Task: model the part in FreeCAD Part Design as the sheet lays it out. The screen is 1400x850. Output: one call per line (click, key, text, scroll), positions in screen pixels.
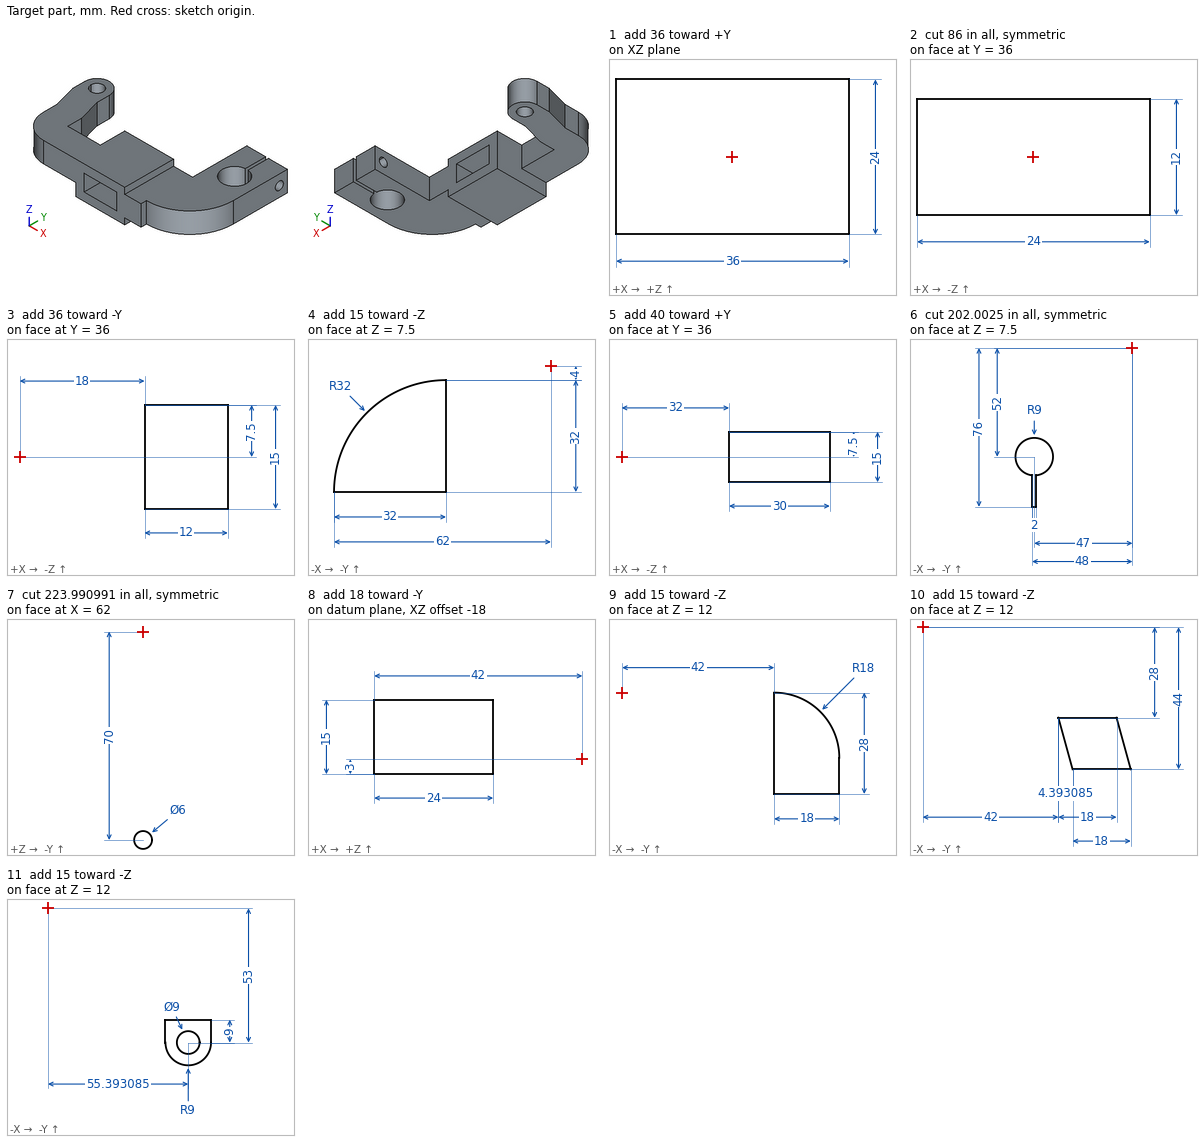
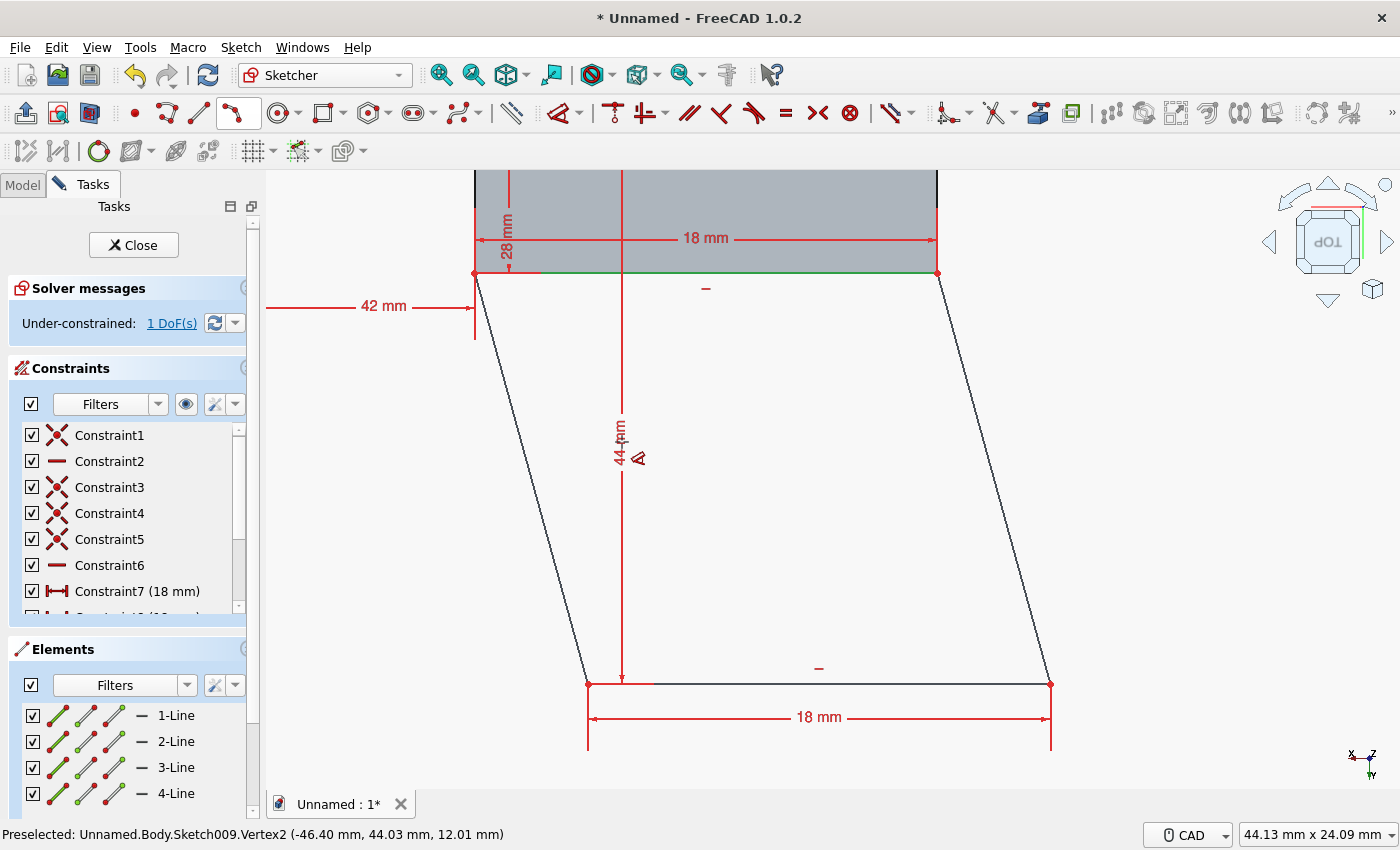
click(509, 396)
click(531, 718)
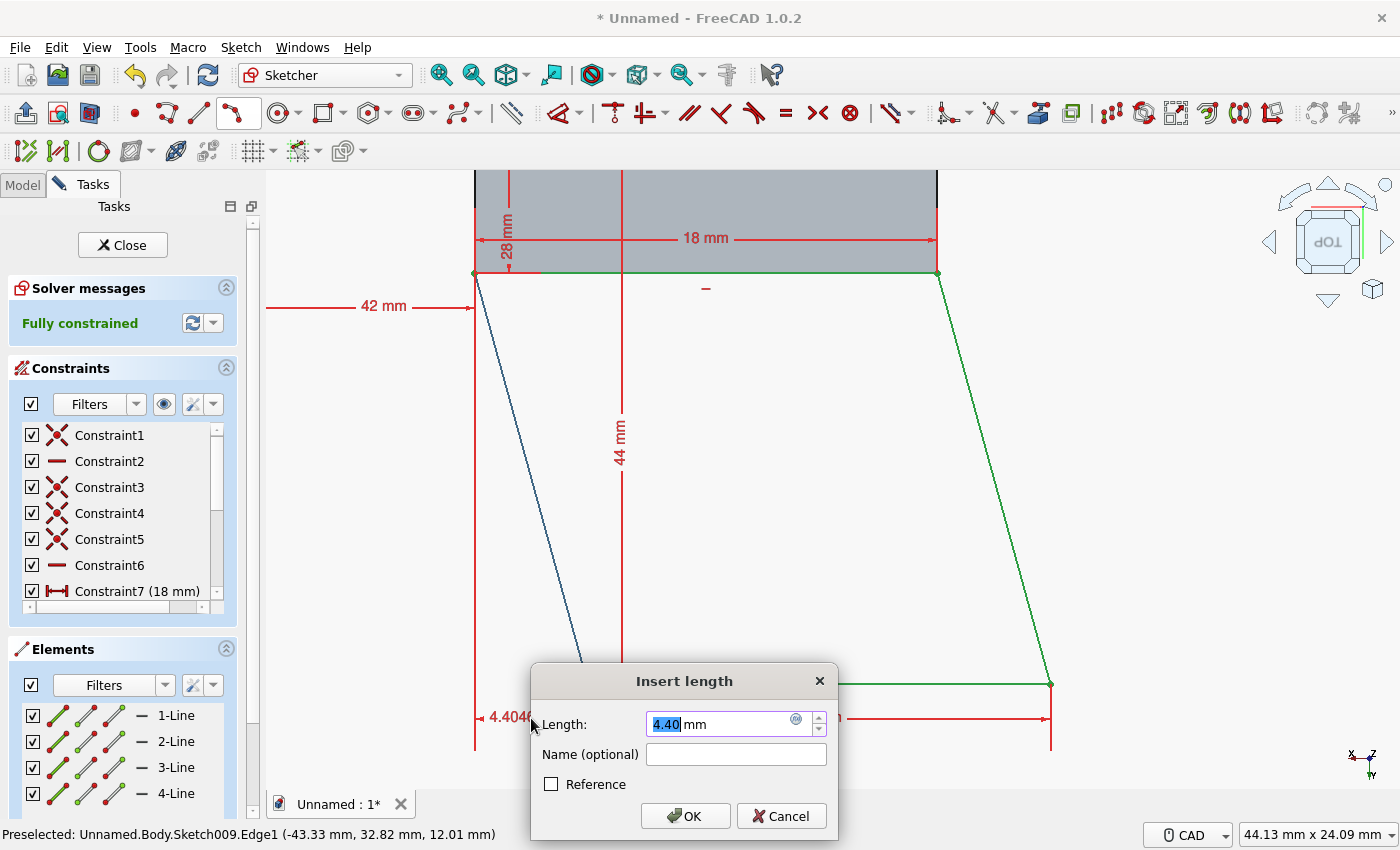
text(4.393085)
key(Return)
key(Escape)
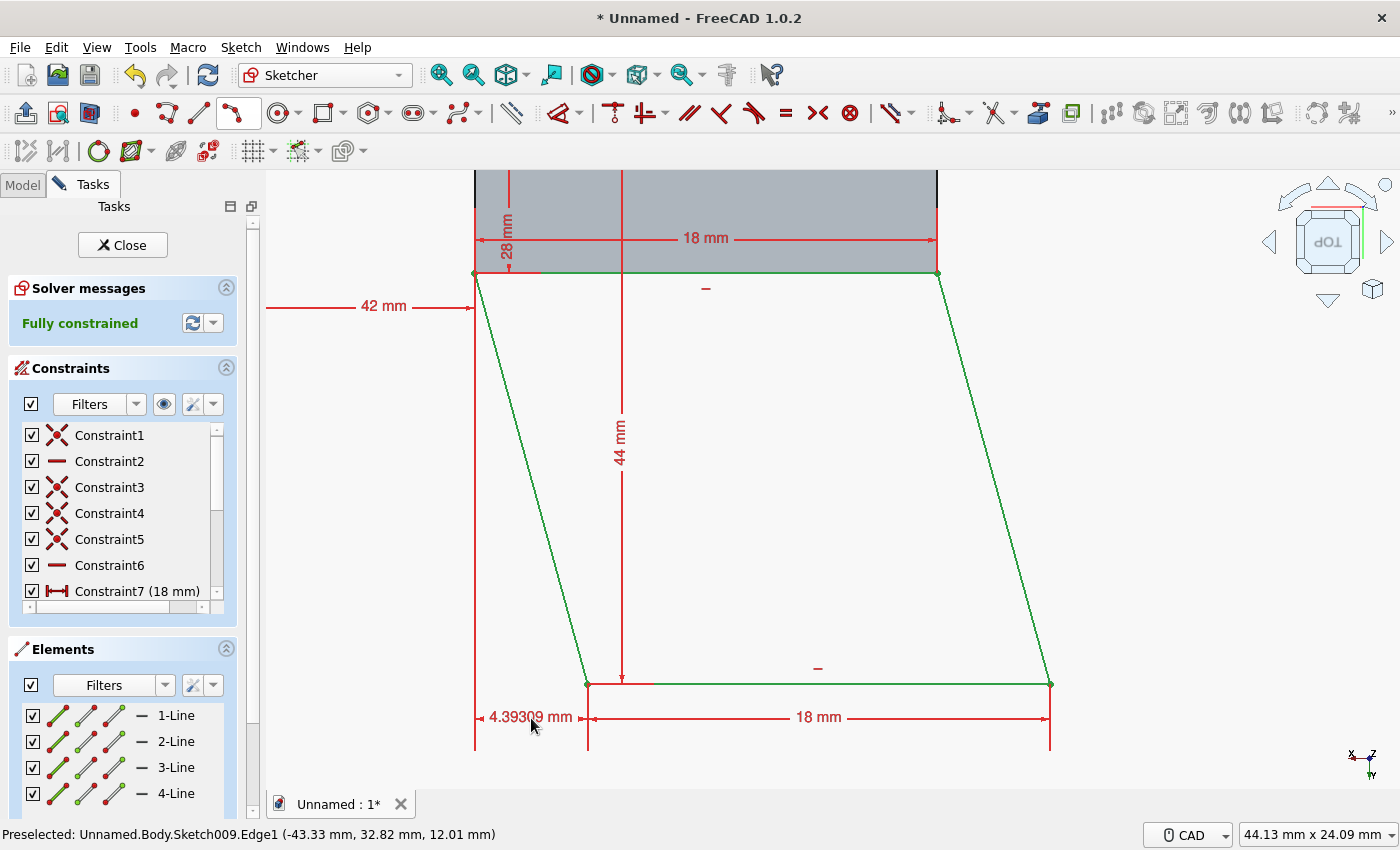
click(123, 245)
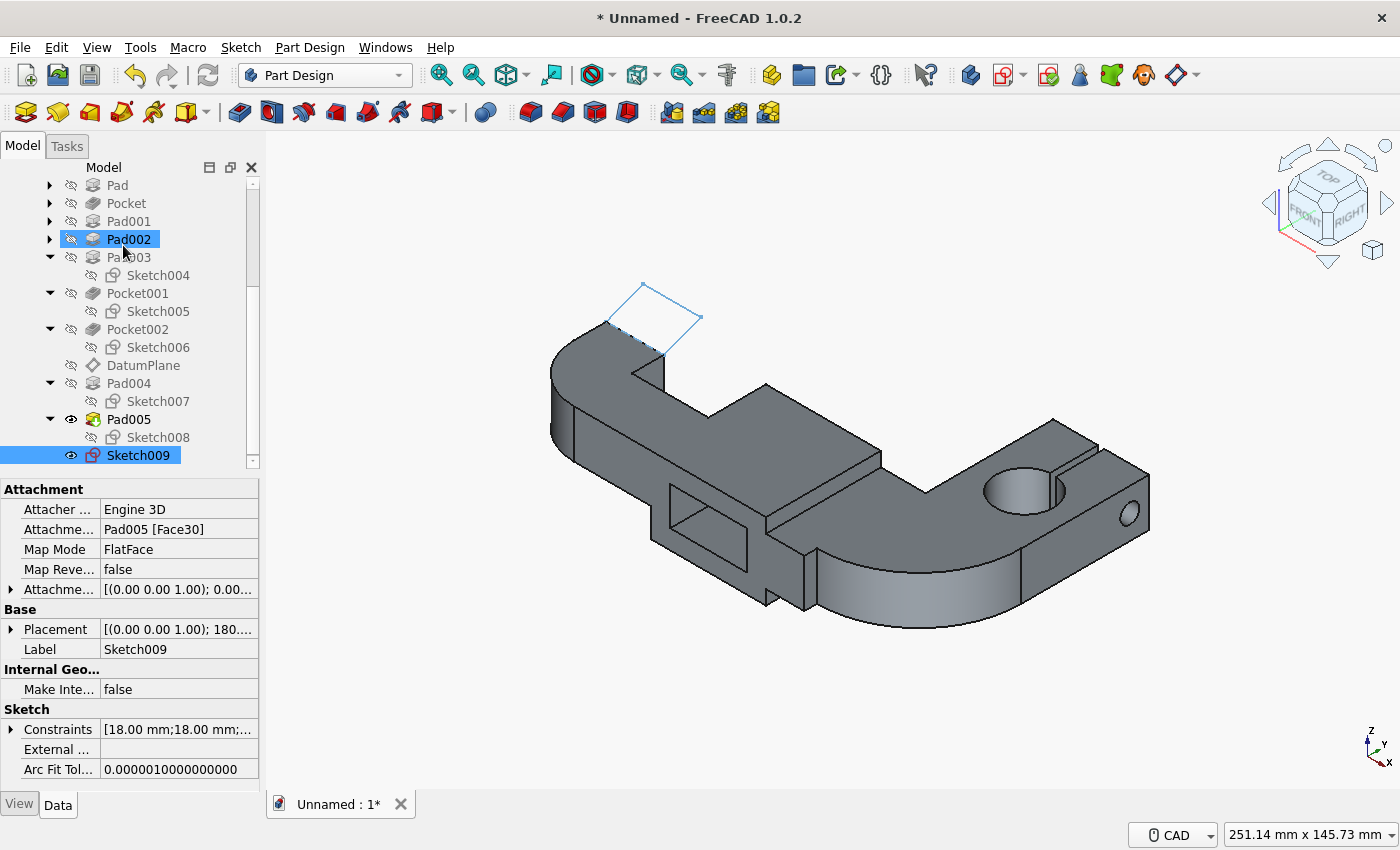
click(26, 112)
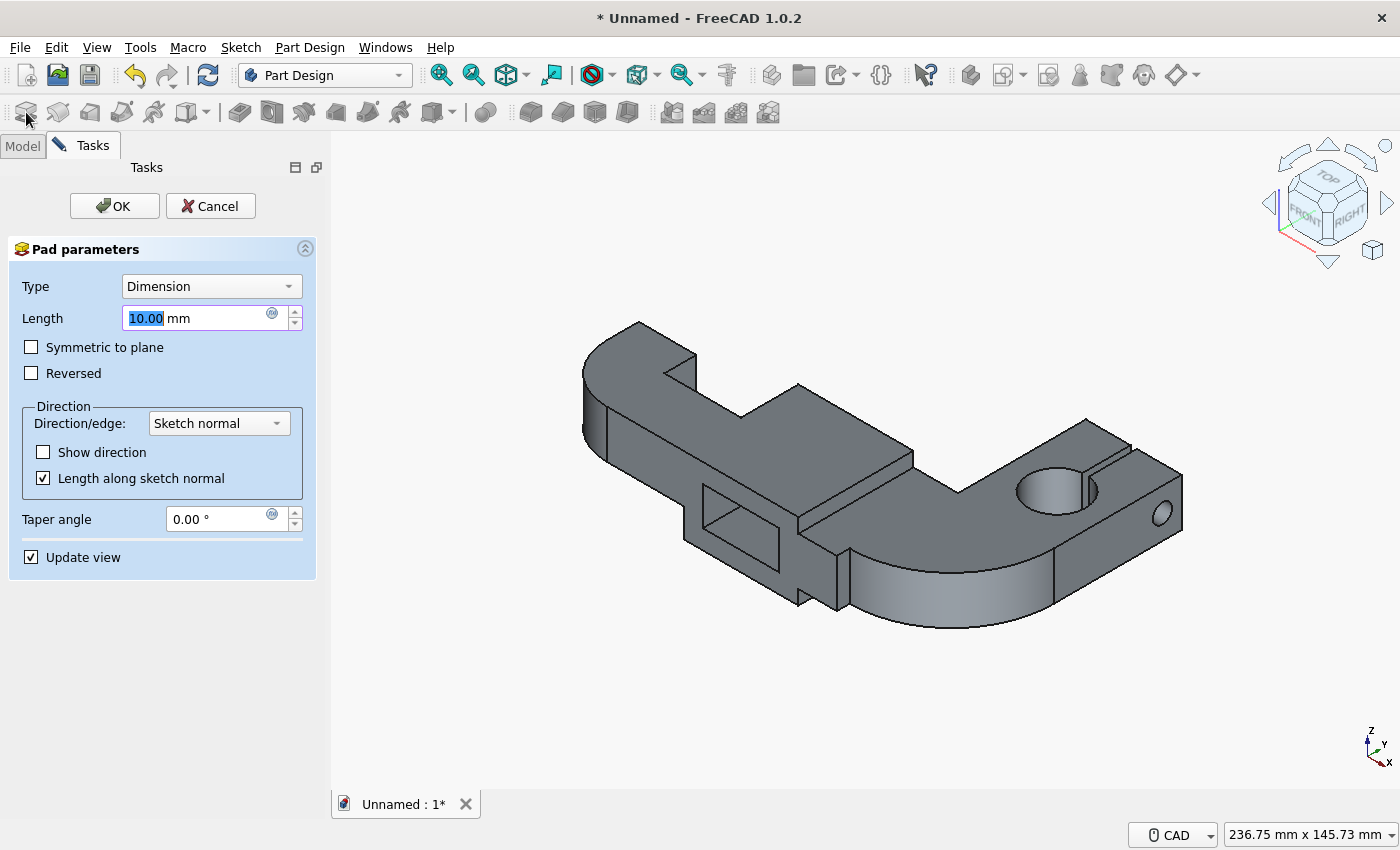
text(15)
key(Tab)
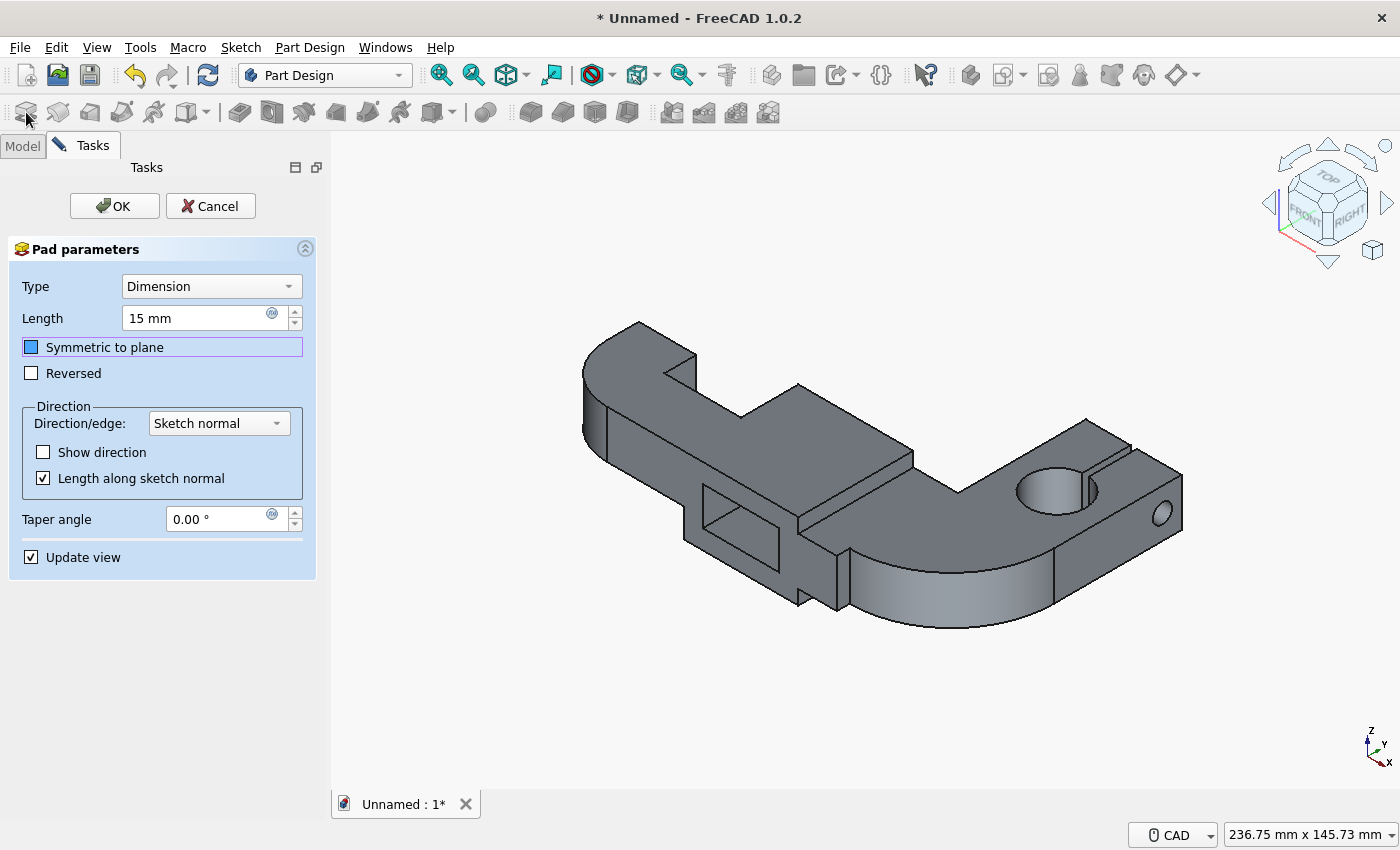
click(30, 373)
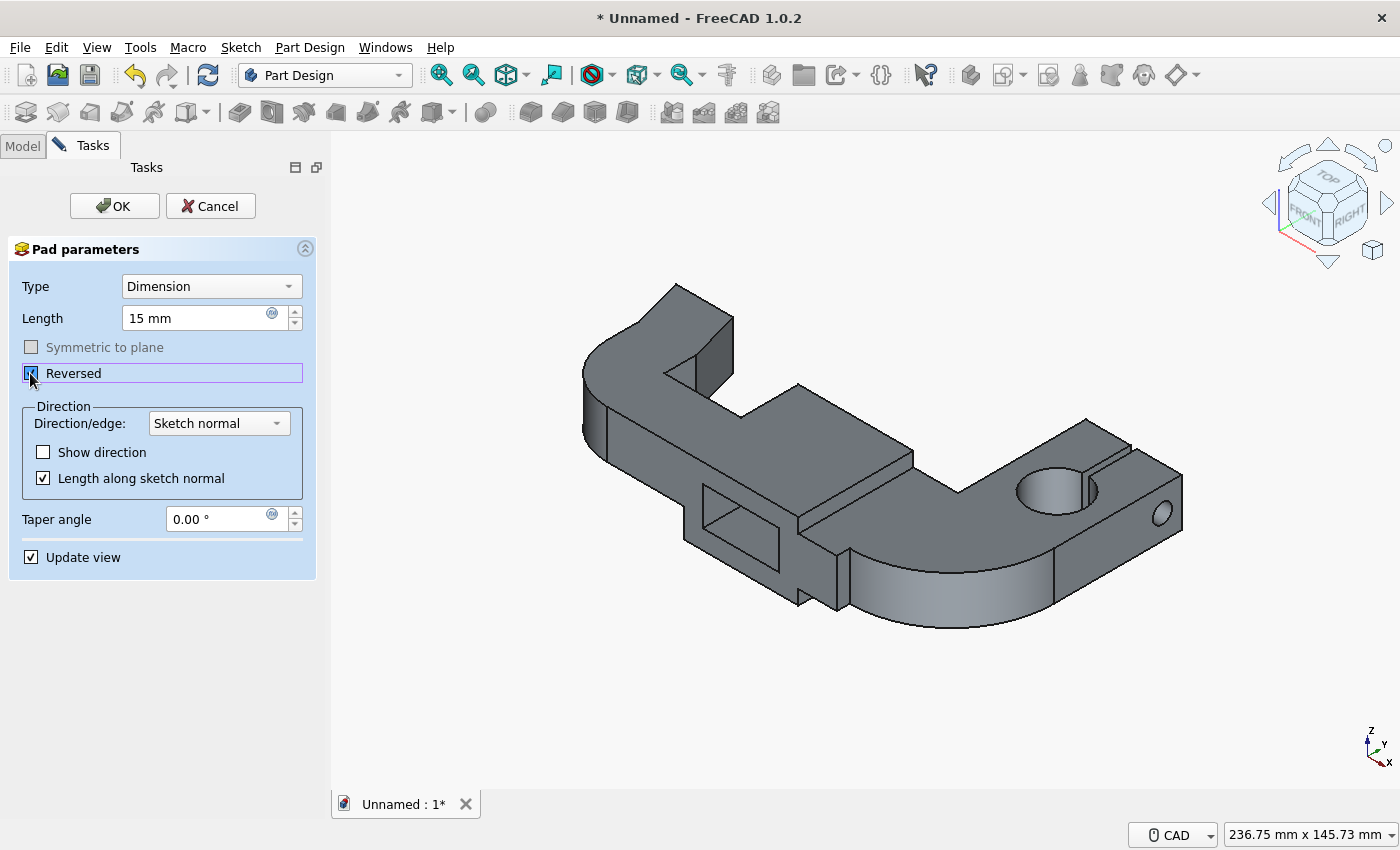
click(115, 206)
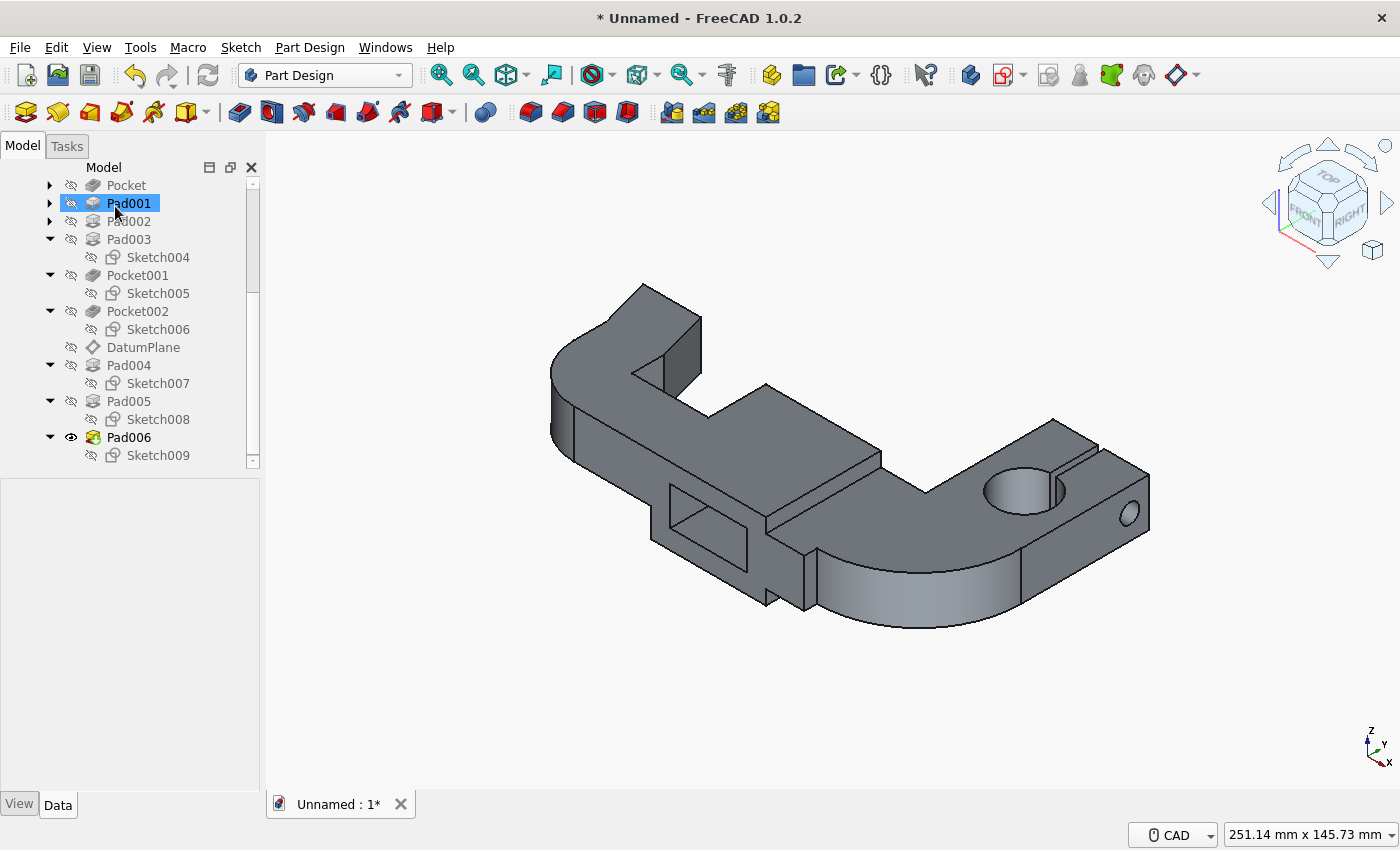
click(760, 455)